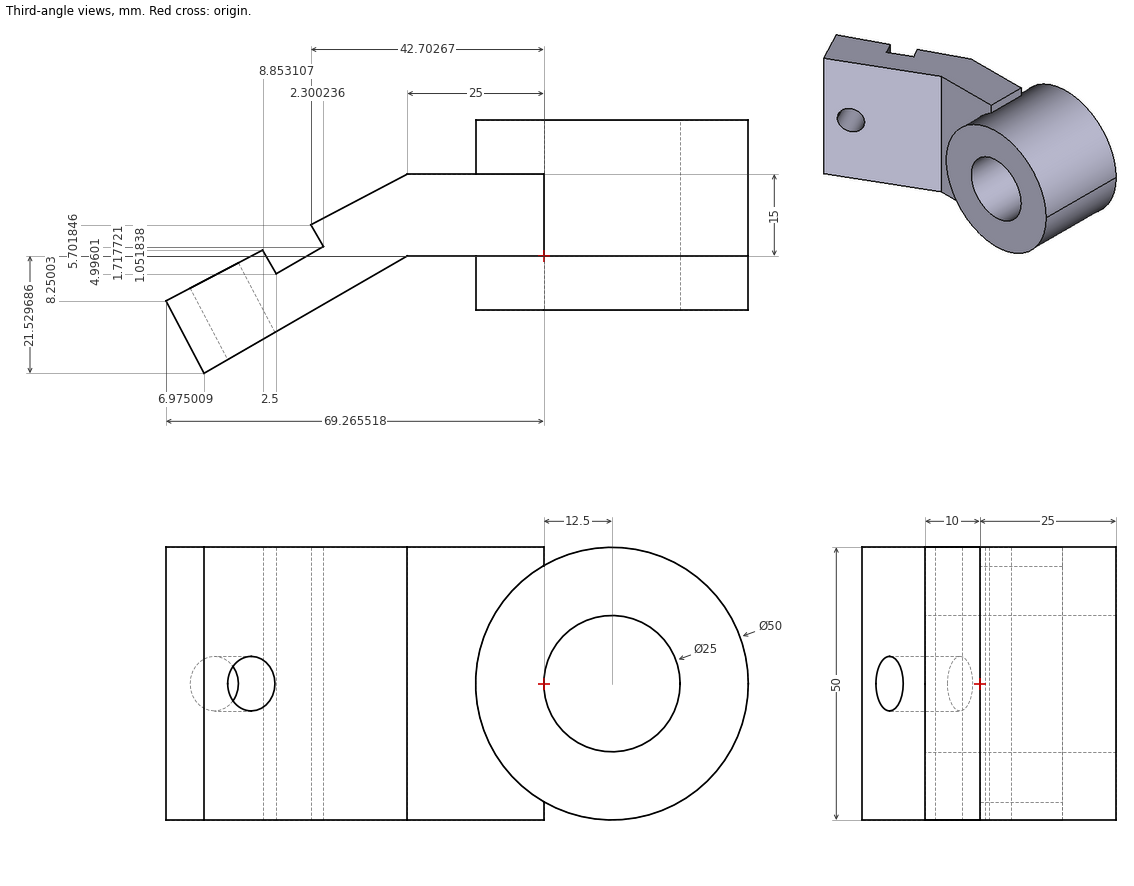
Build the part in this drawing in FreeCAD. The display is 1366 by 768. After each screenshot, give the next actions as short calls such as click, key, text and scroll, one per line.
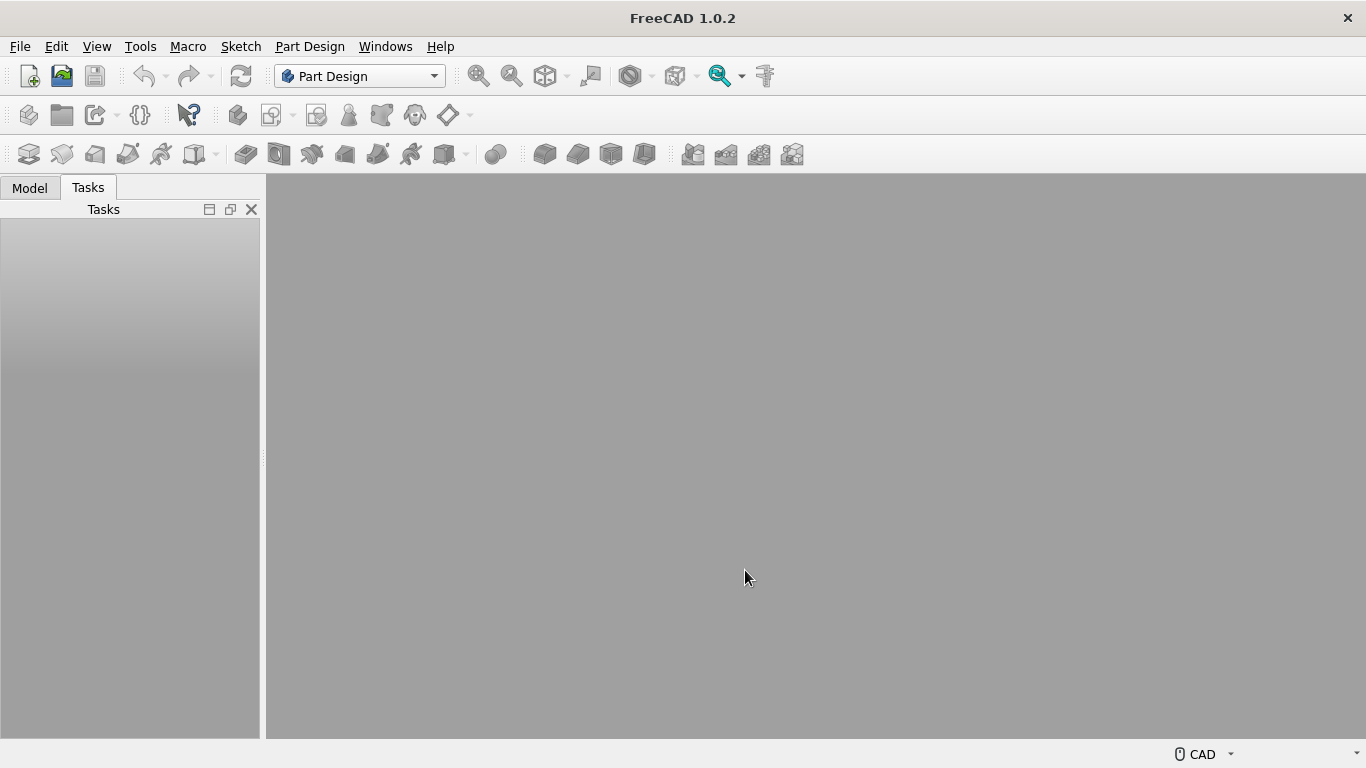
key(ctrl+n)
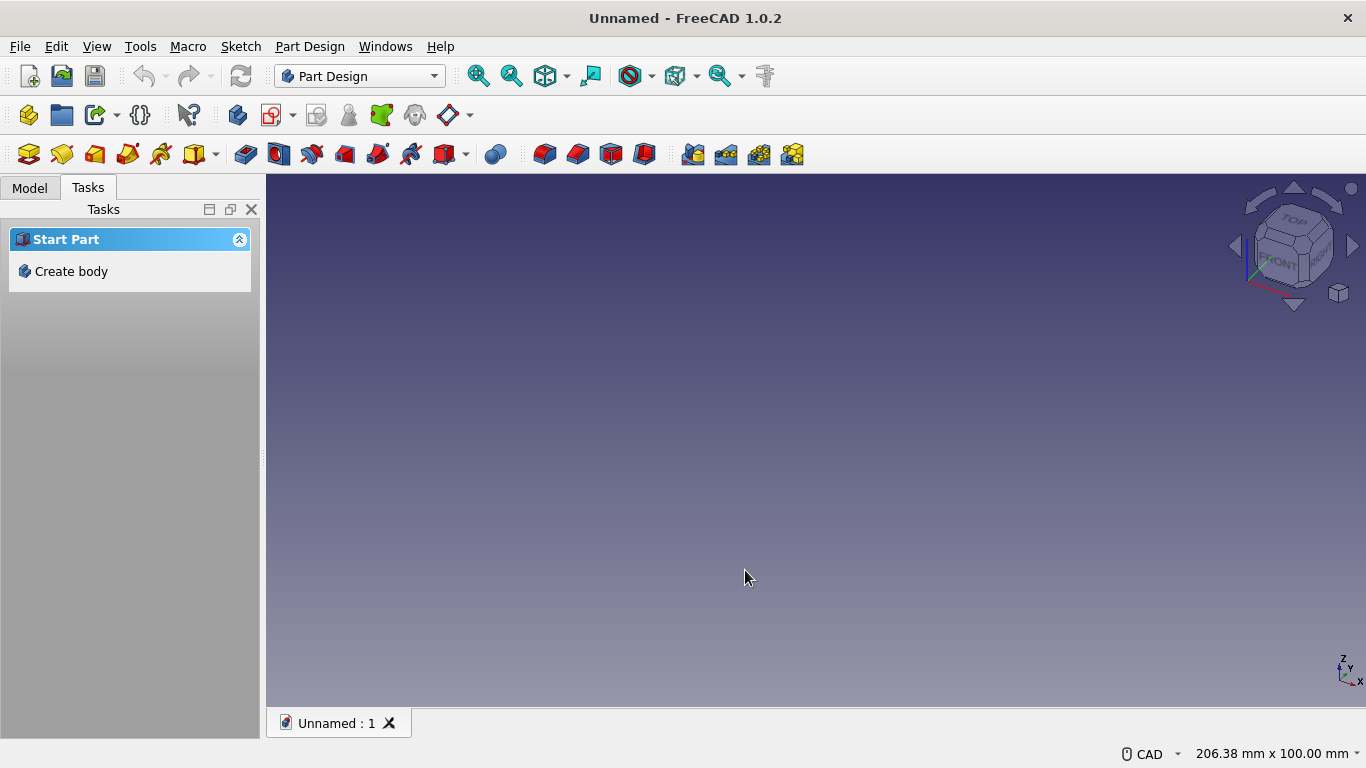
click(270, 116)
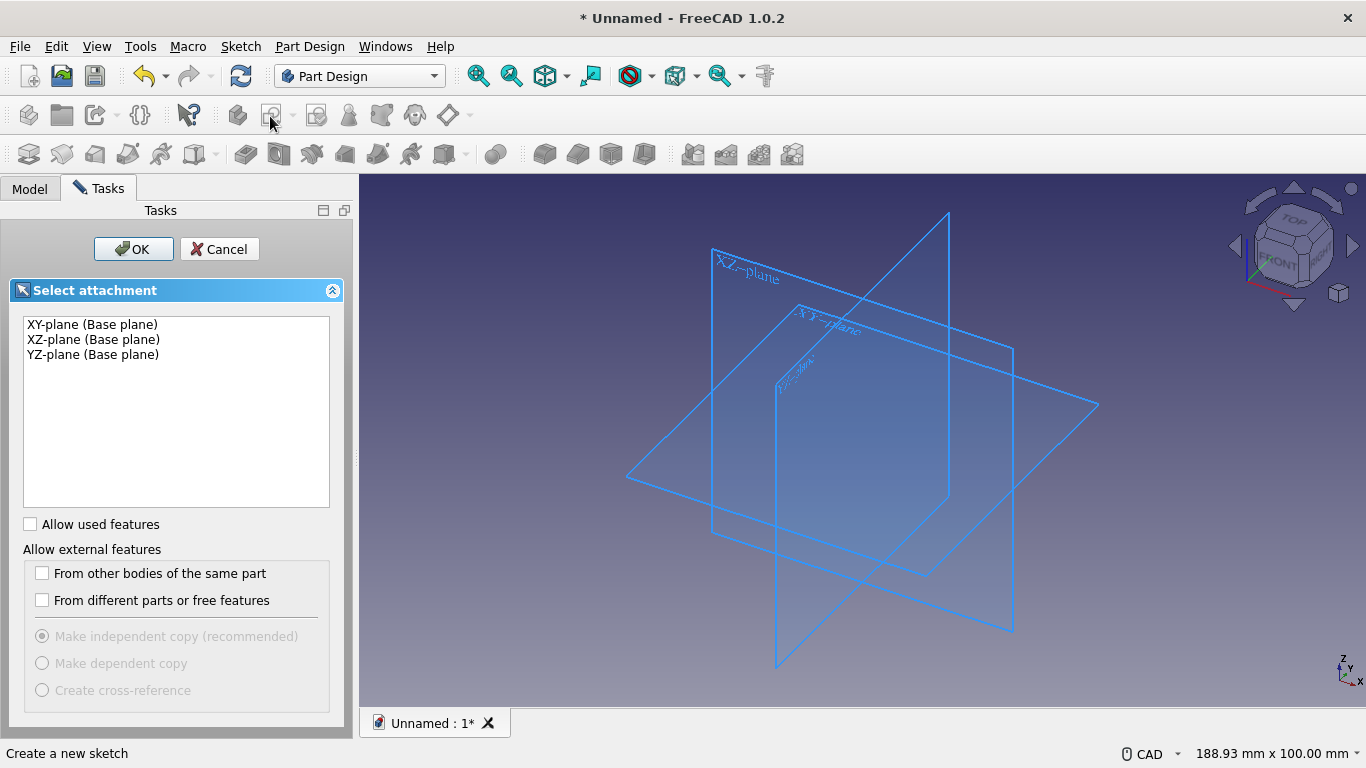
click(84, 324)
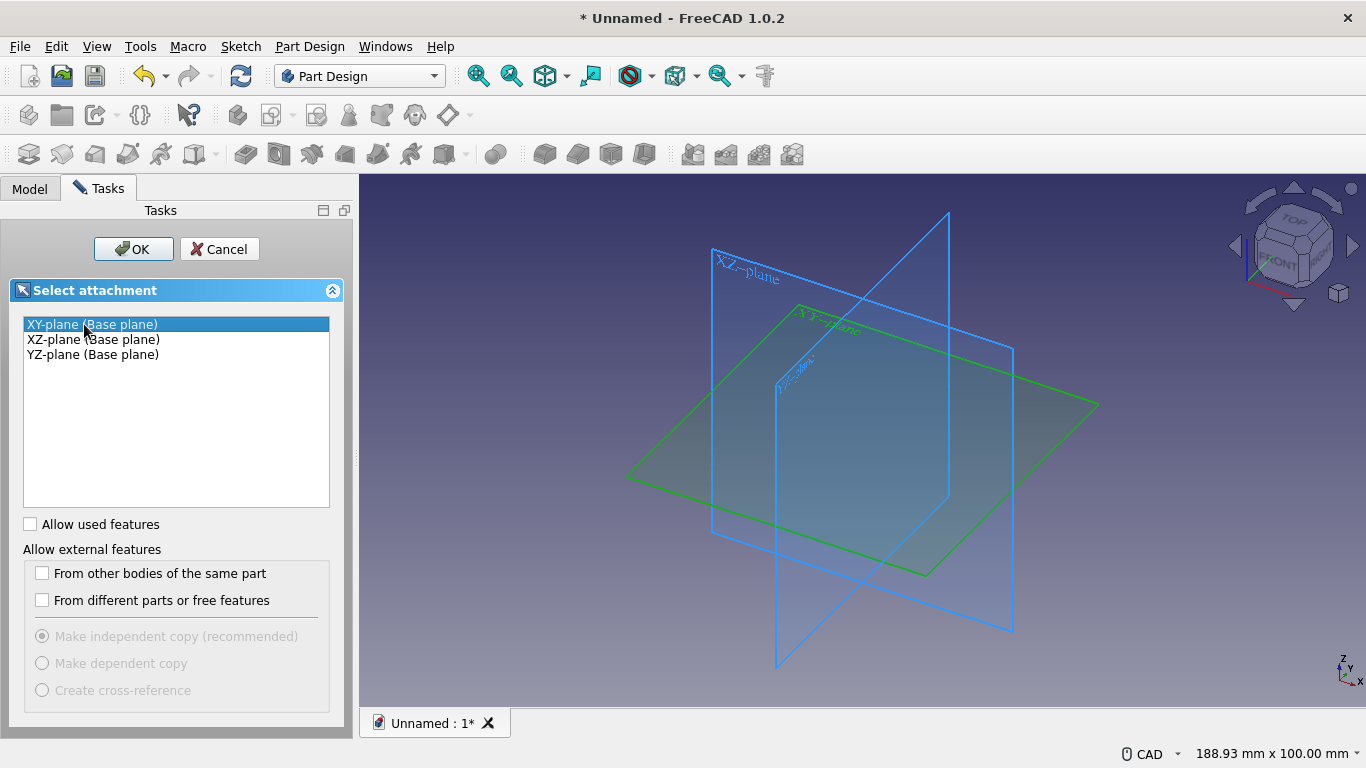
click(134, 249)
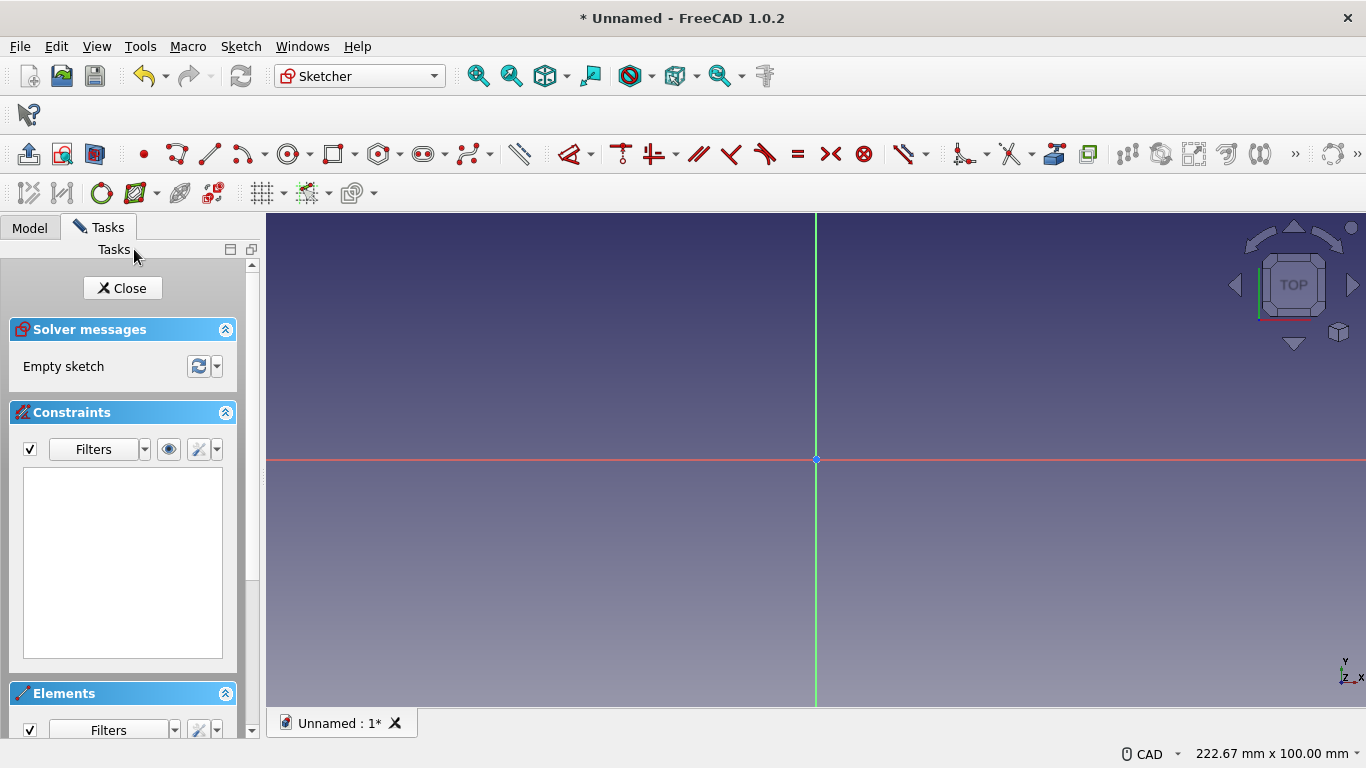
scroll(520, 496, up, 3)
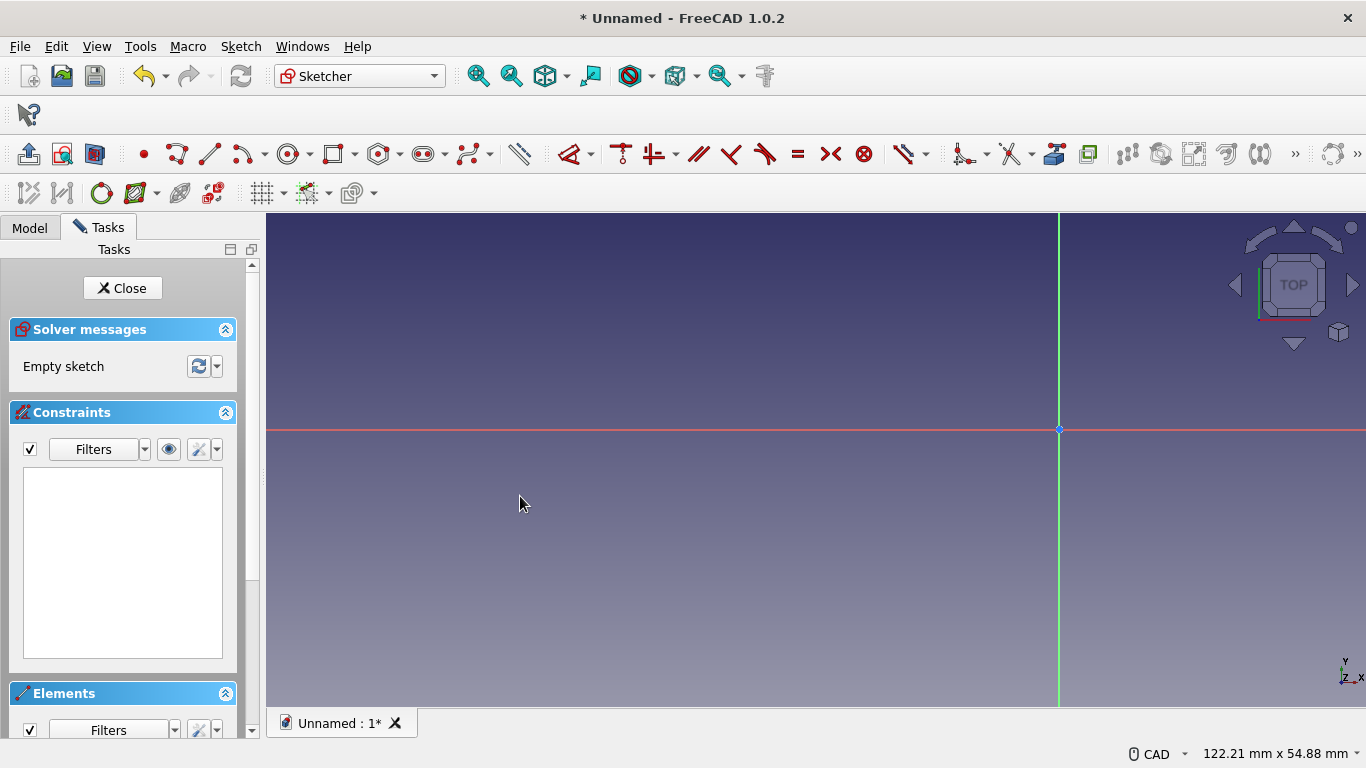
click(177, 154)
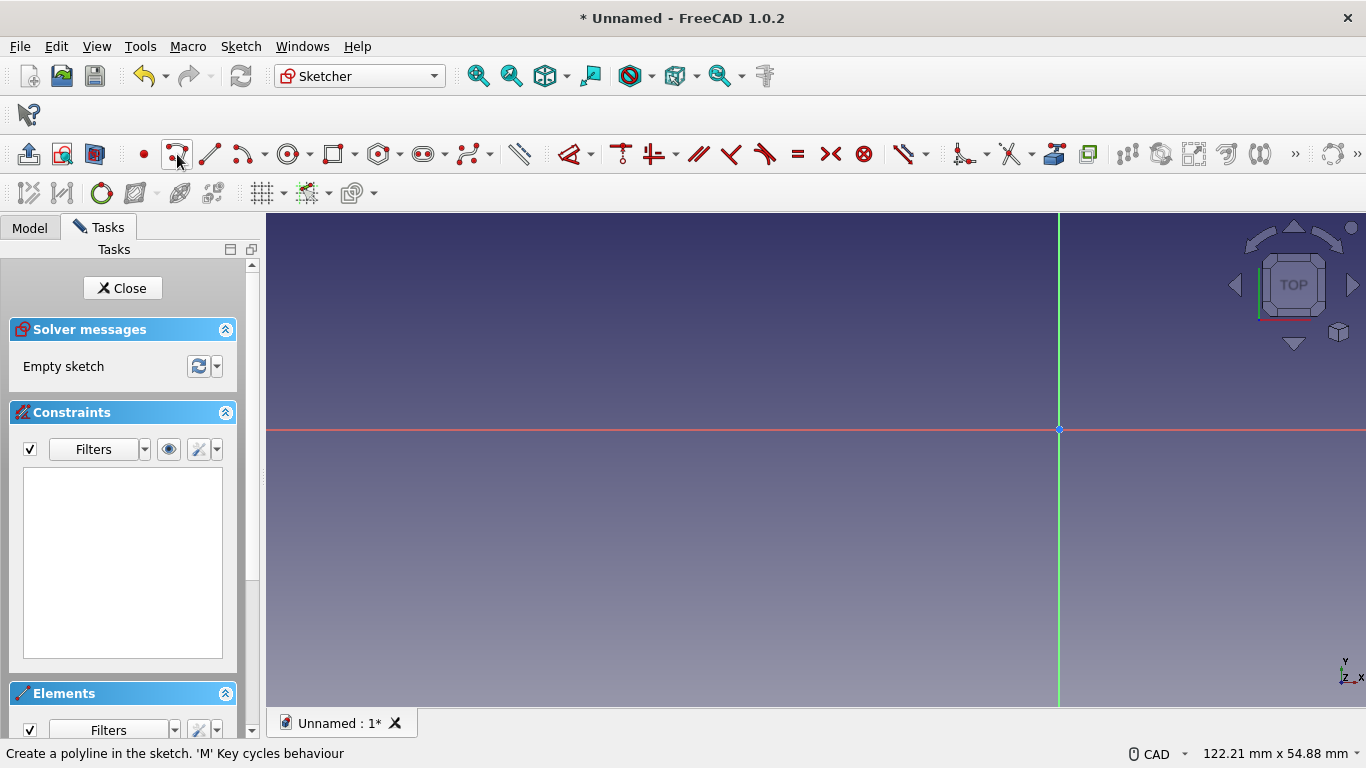
click(1059, 430)
click(1050, 295)
click(834, 295)
click(436, 504)
click(498, 624)
click(834, 439)
click(1059, 430)
key(Escape)
key(Escape)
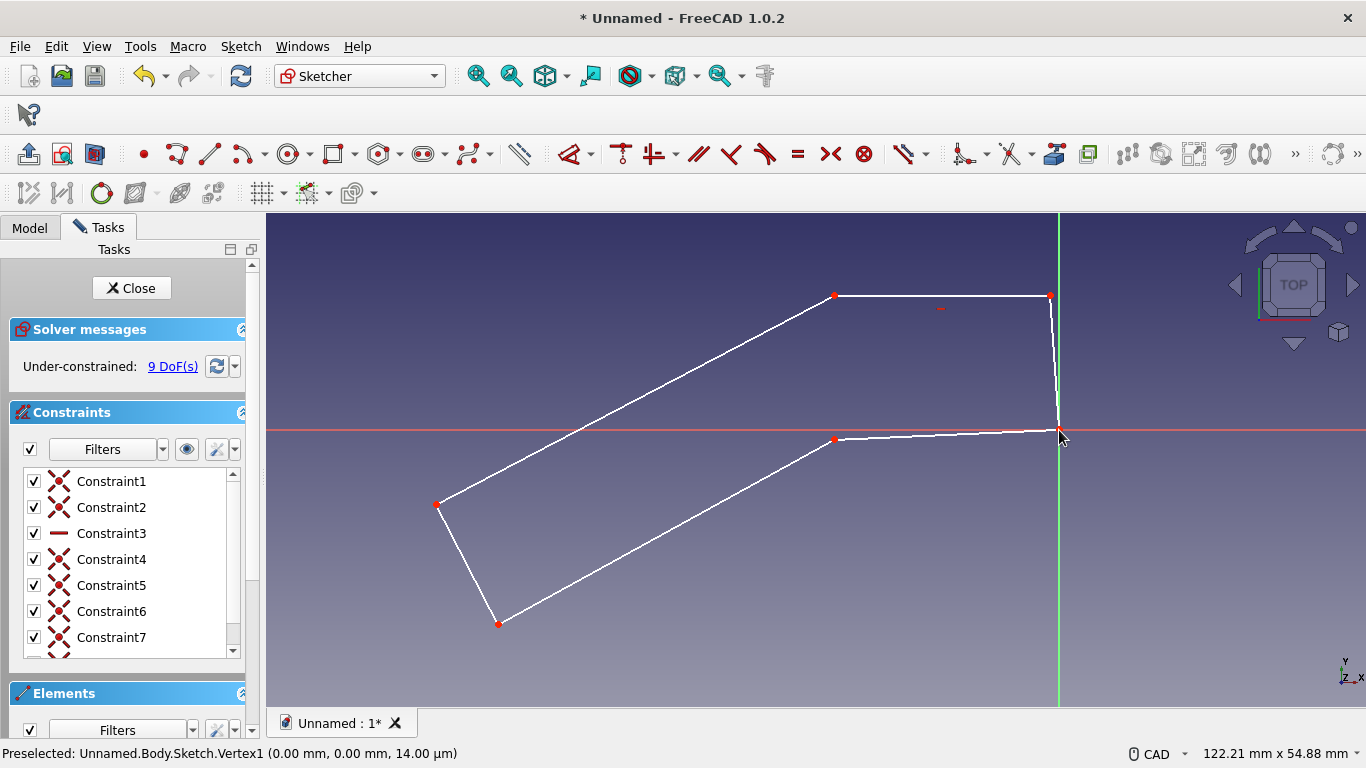
click(1056, 390)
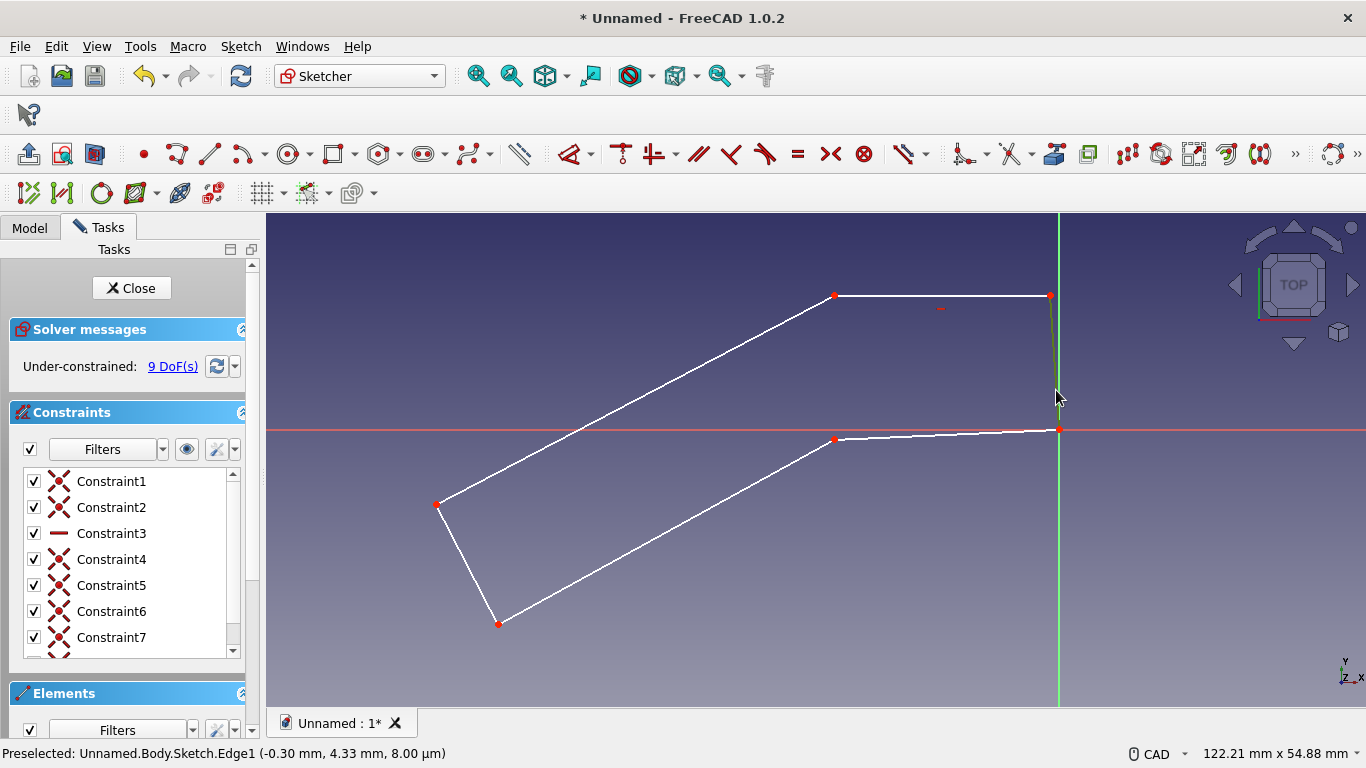
key(v)